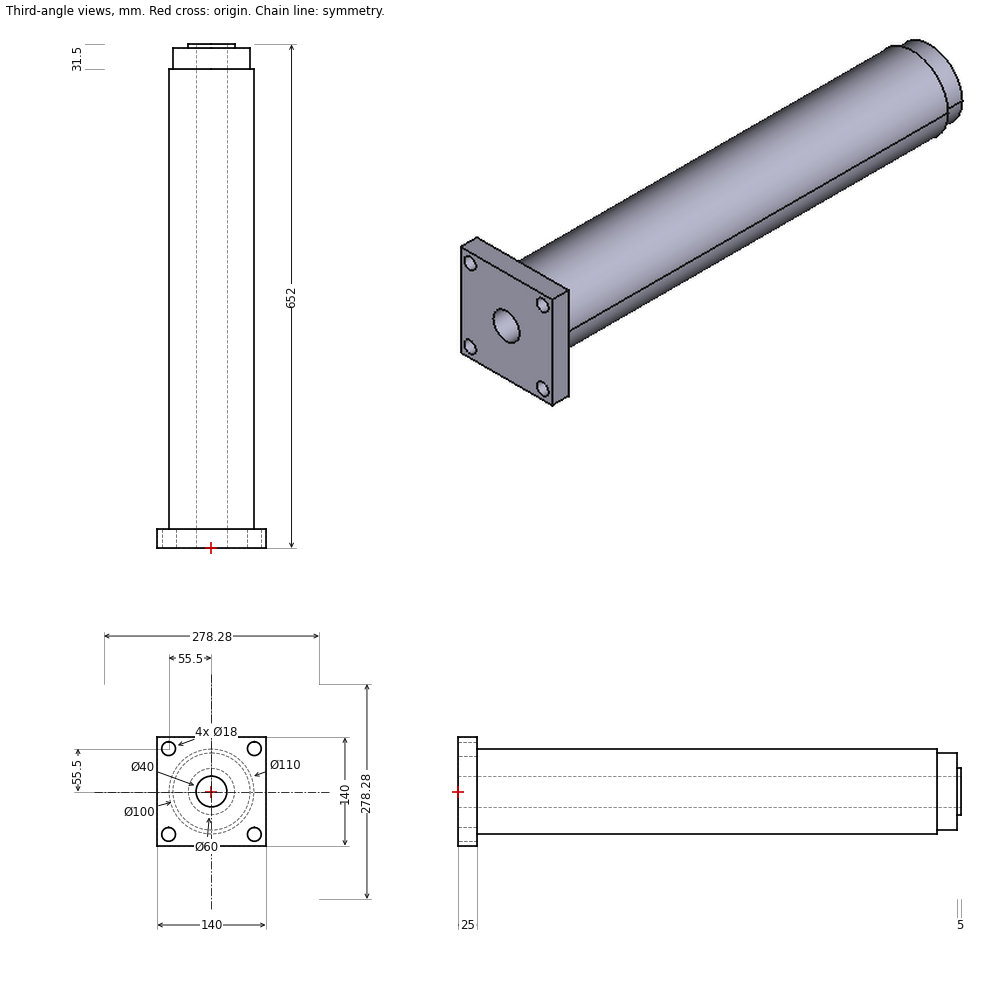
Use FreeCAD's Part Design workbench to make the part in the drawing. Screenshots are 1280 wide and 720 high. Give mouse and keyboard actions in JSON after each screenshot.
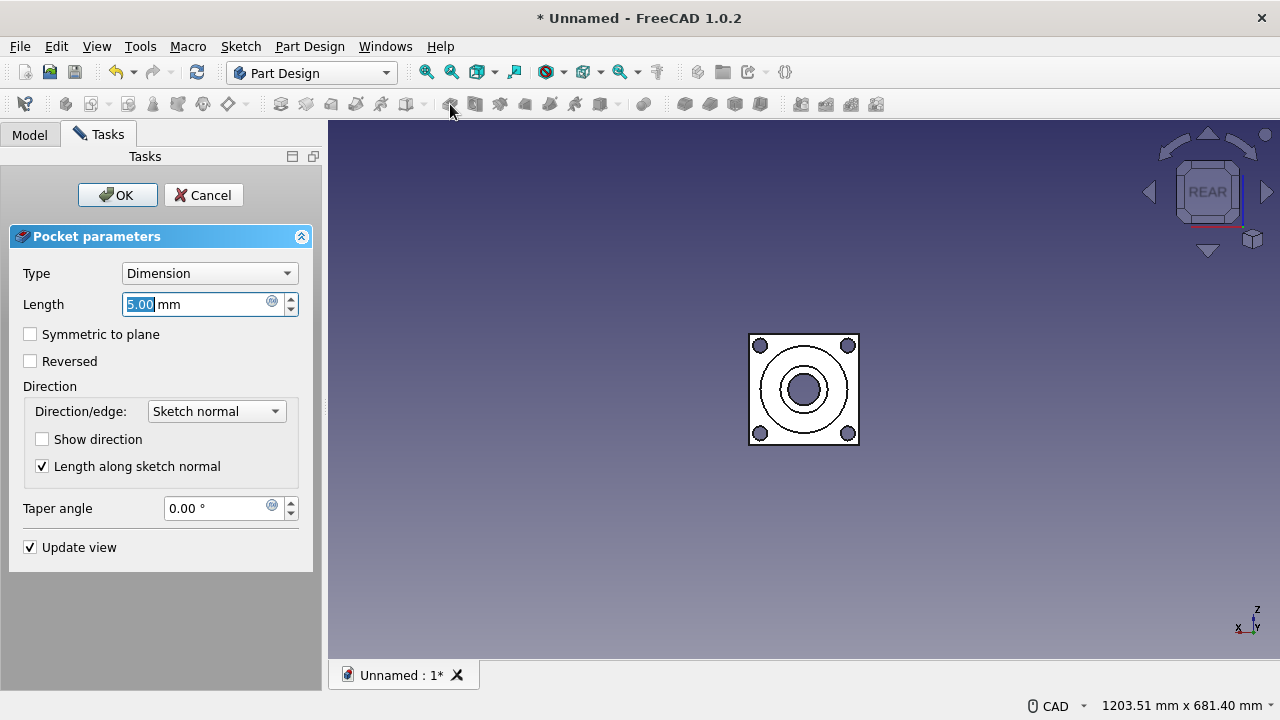
{"action": "type", "text": "5"}
{"action": "key", "text": "Tab"}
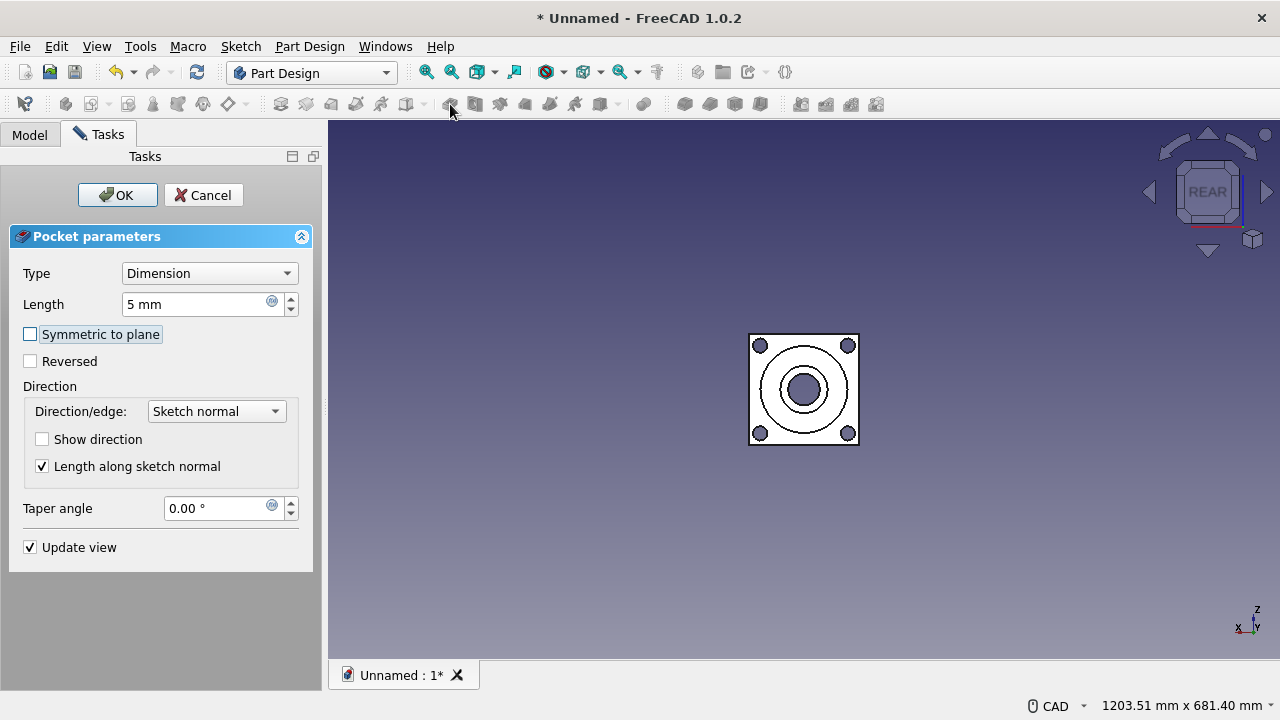
{"action": "left_click", "coordinate": [118, 195]}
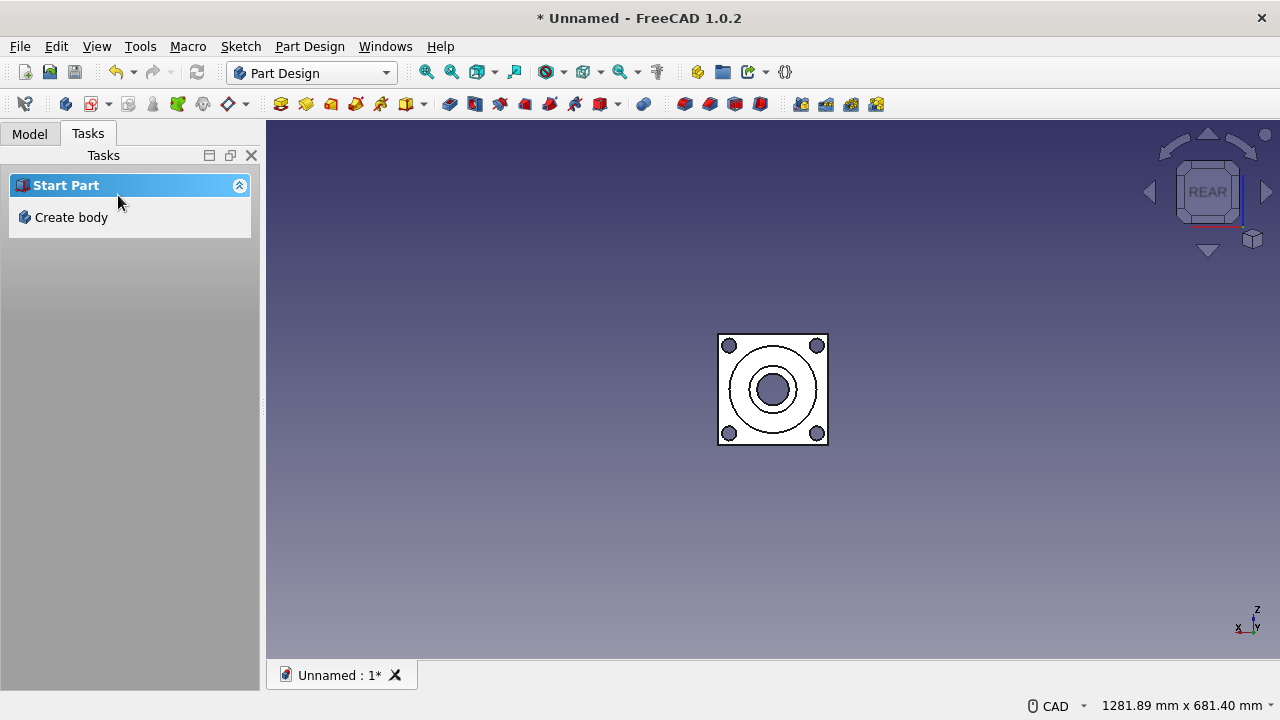
{"action": "left_click", "coordinate": [427, 72]}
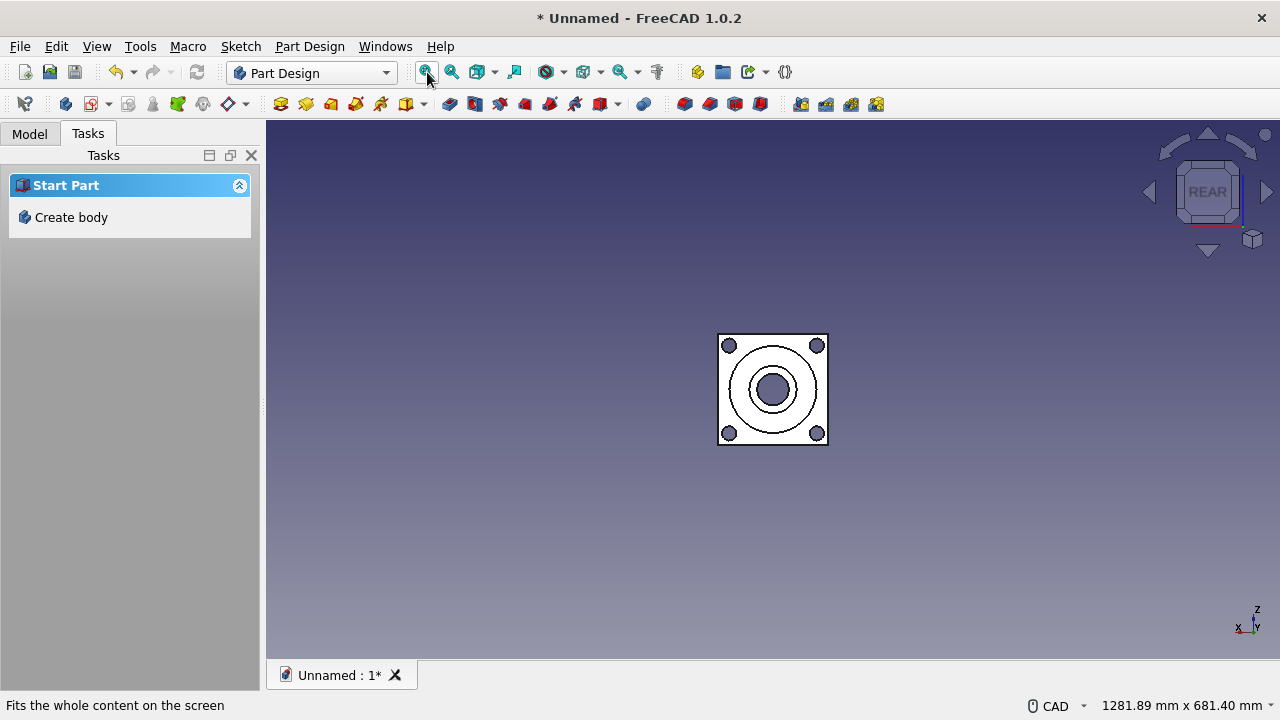
{"action": "scroll", "coordinate": [753, 388], "scroll_direction": "up", "scroll_amount": 7}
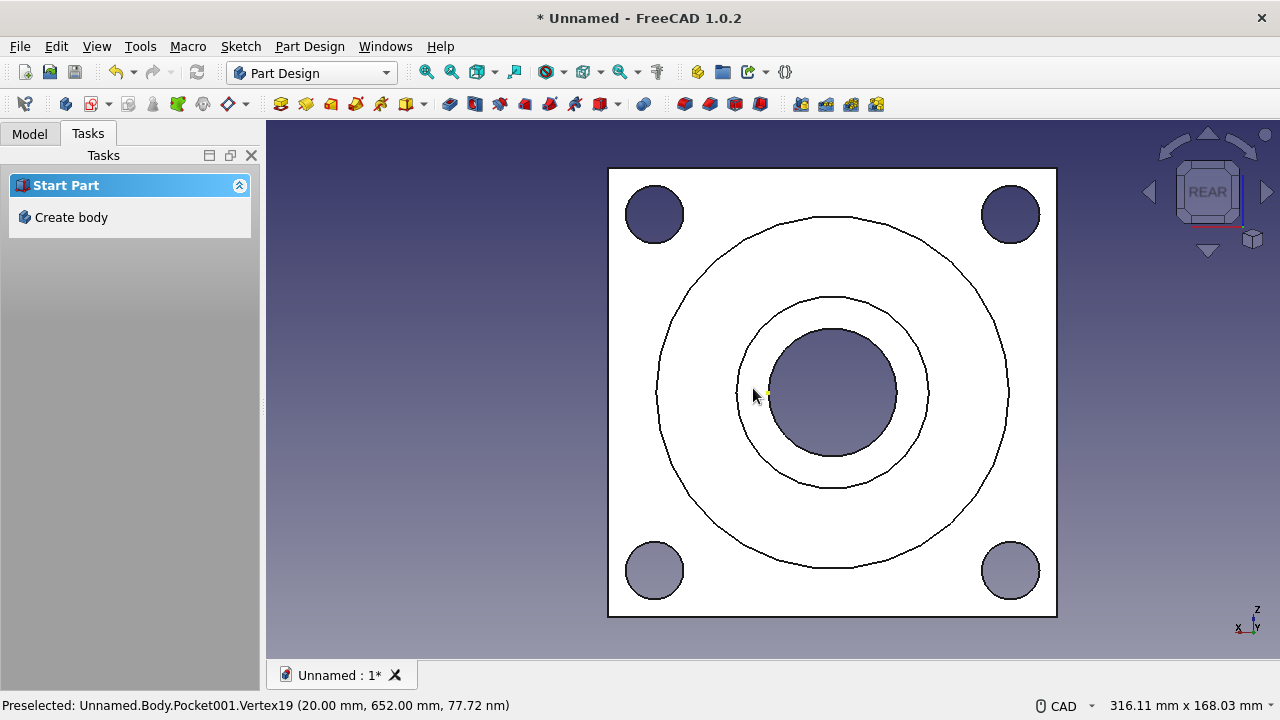
{"action": "left_click", "coordinate": [750, 392]}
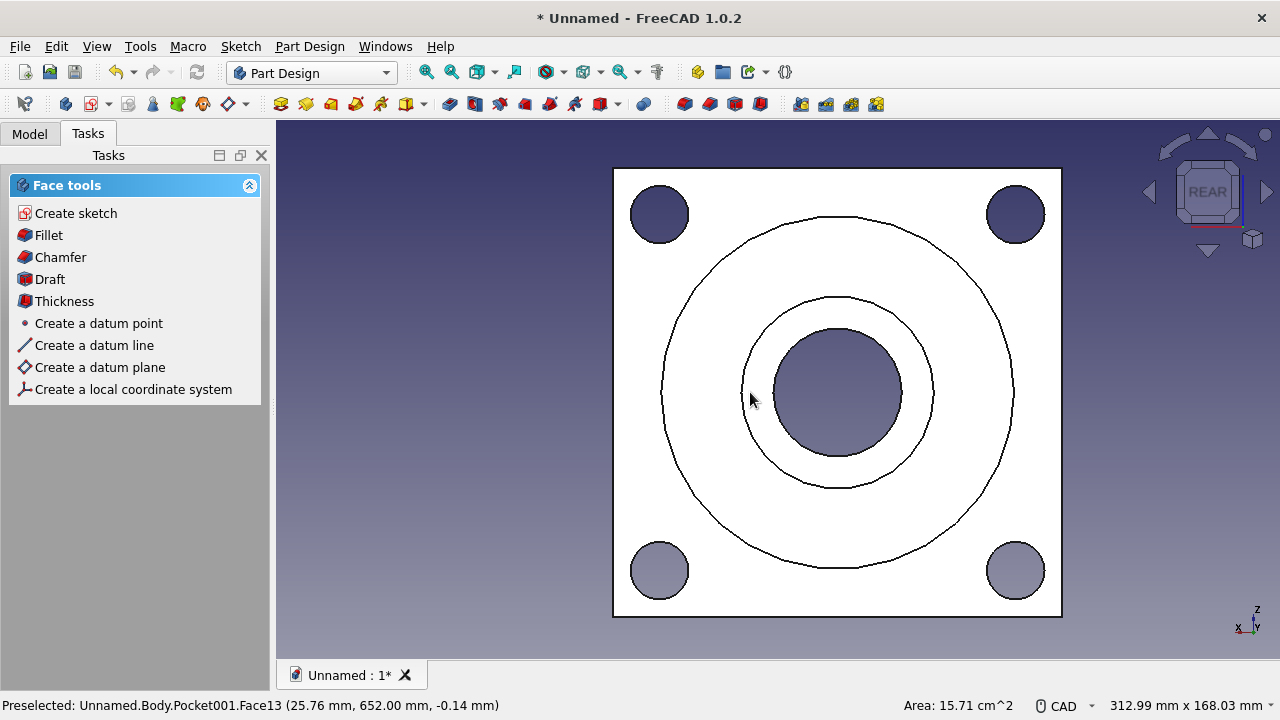
{"action": "left_click", "coordinate": [90, 104]}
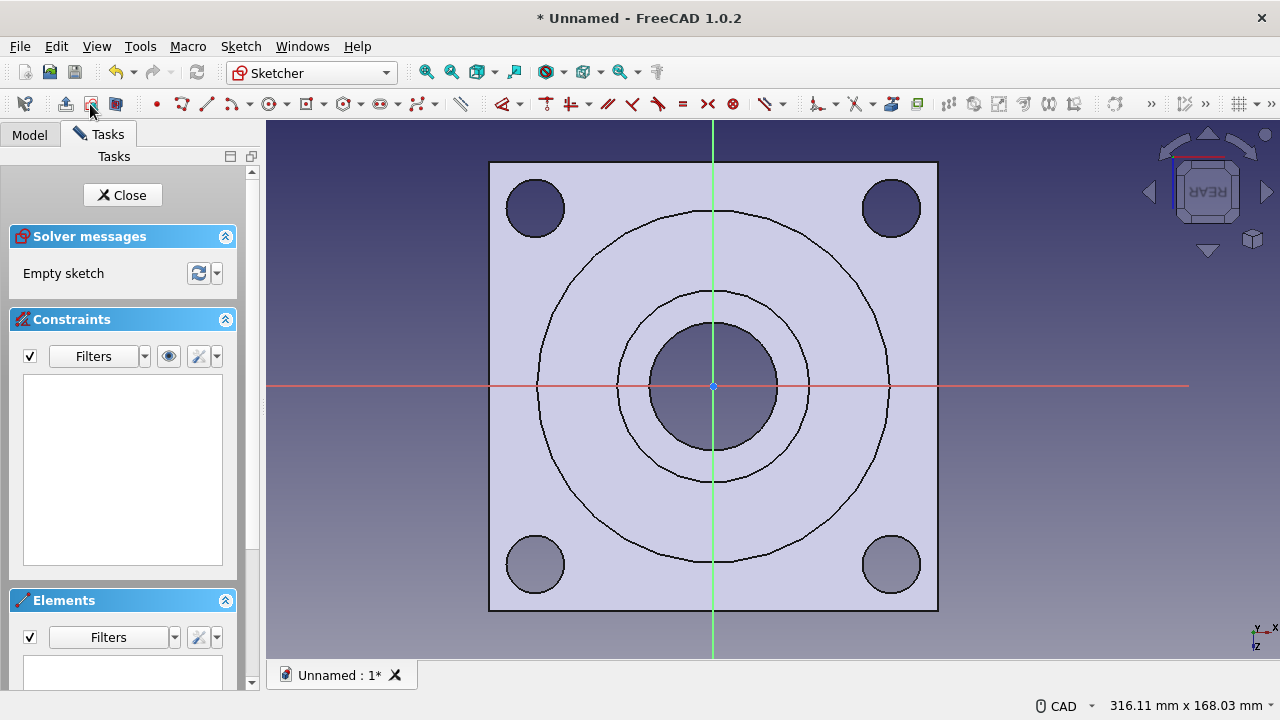
{"action": "scroll", "coordinate": [699, 391], "scroll_direction": "down", "scroll_amount": 5}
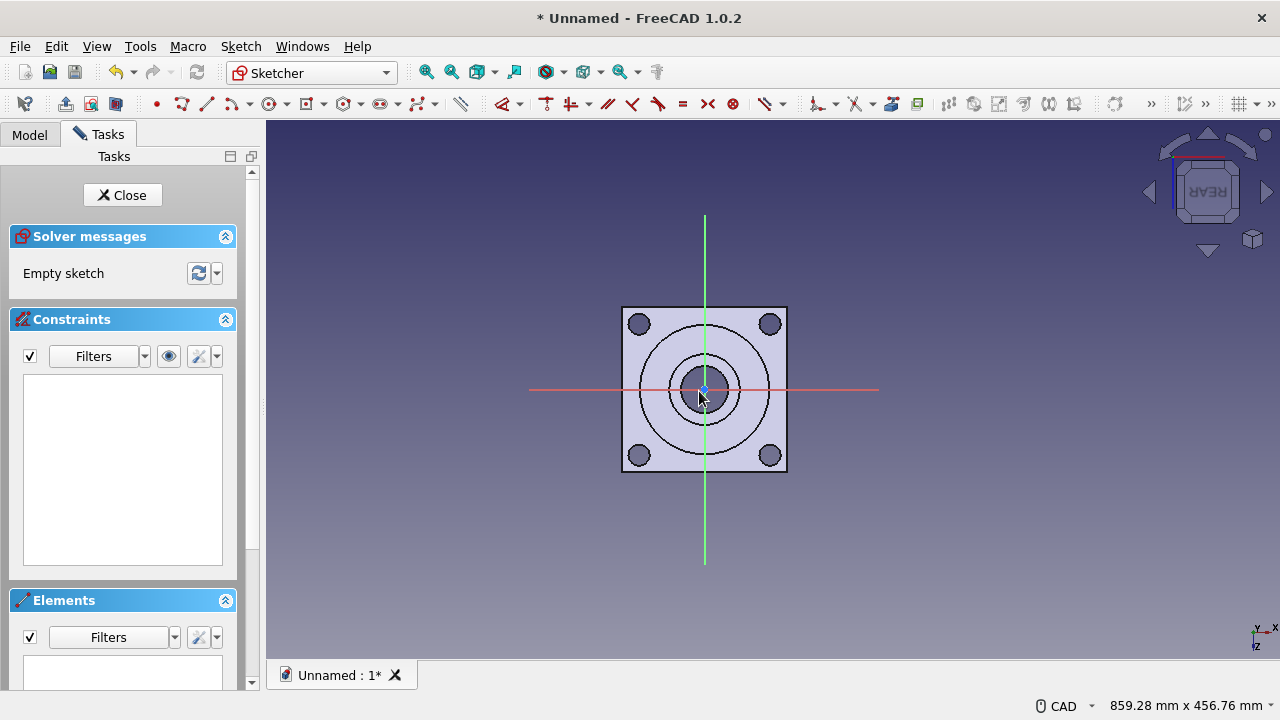
{"action": "left_click", "coordinate": [306, 104]}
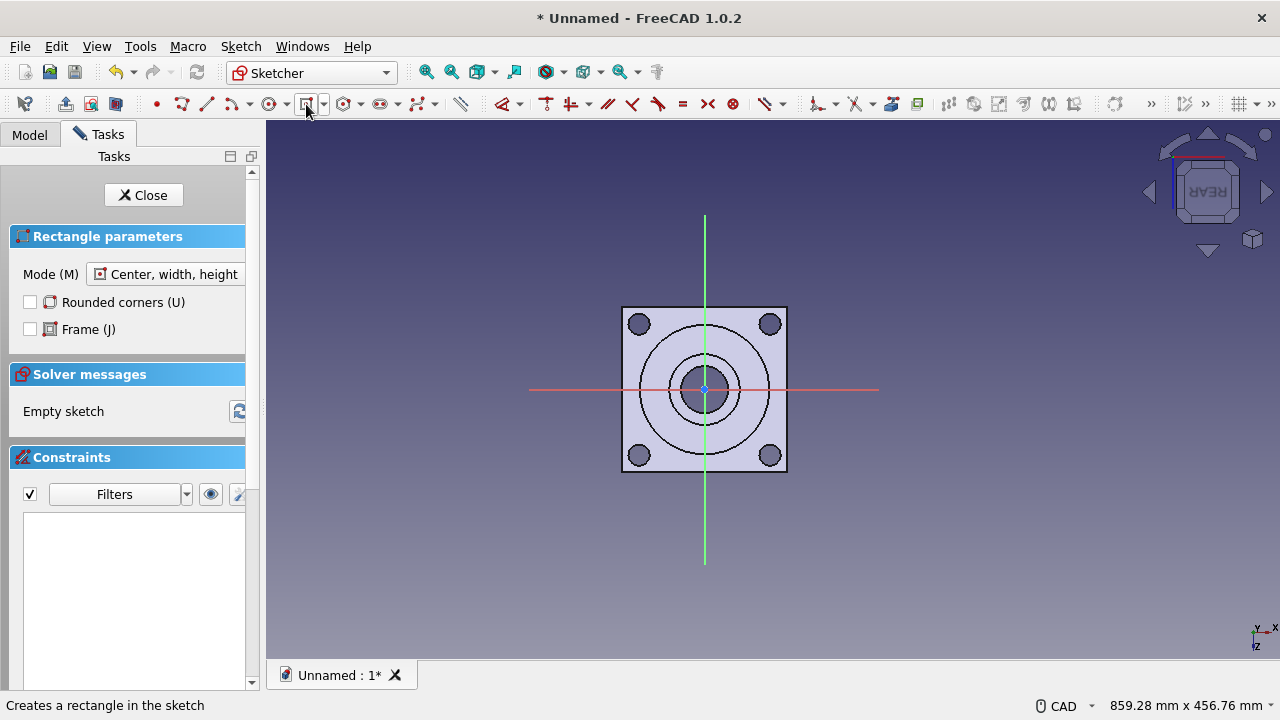
{"action": "left_click", "coordinate": [705, 390]}
{"action": "mouse_move", "coordinate": [869, 225]}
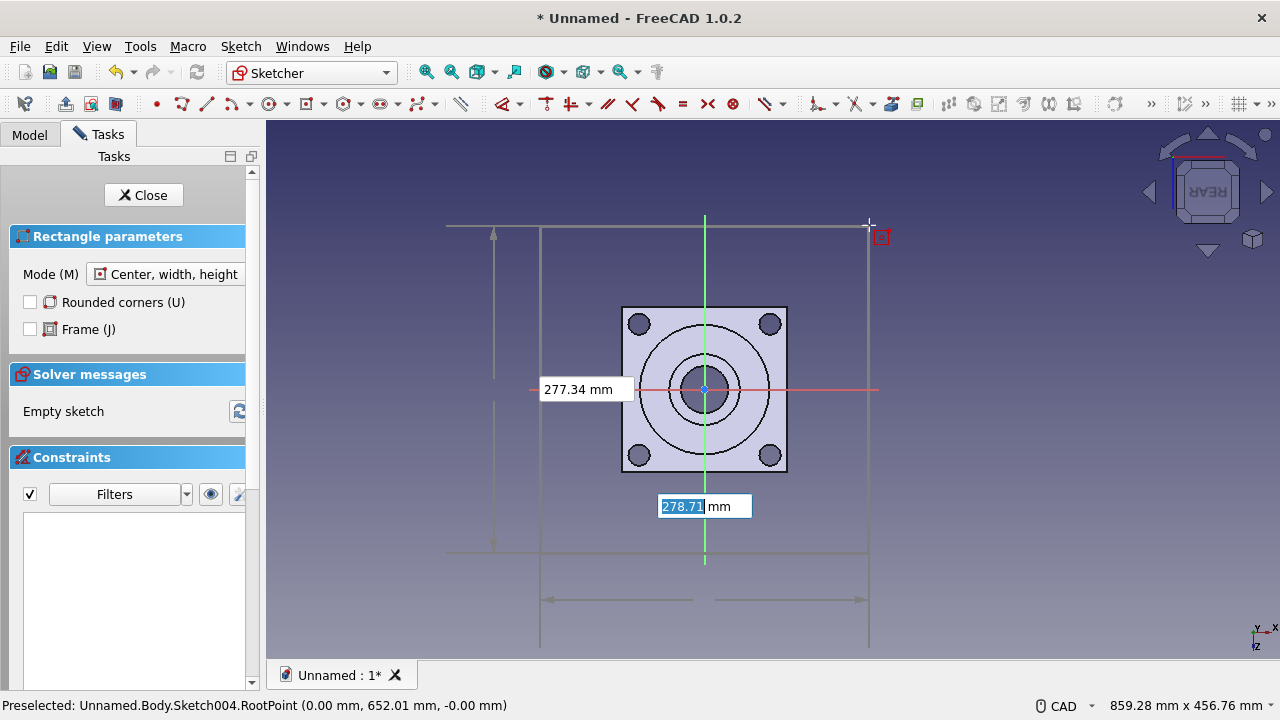
{"action": "type", "text": "278.28"}
{"action": "key", "text": "Tab"}
{"action": "type", "text": "278.28"}
{"action": "key", "text": "Return"}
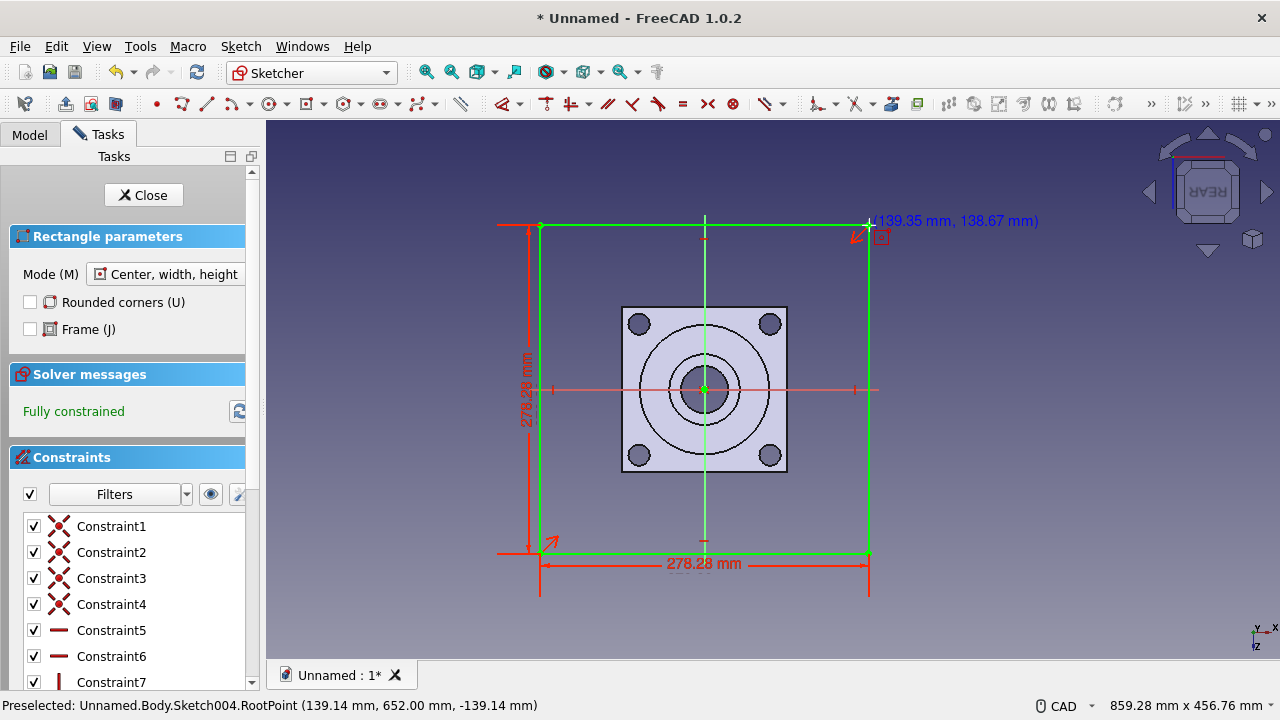
{"action": "left_click", "coordinate": [268, 104]}